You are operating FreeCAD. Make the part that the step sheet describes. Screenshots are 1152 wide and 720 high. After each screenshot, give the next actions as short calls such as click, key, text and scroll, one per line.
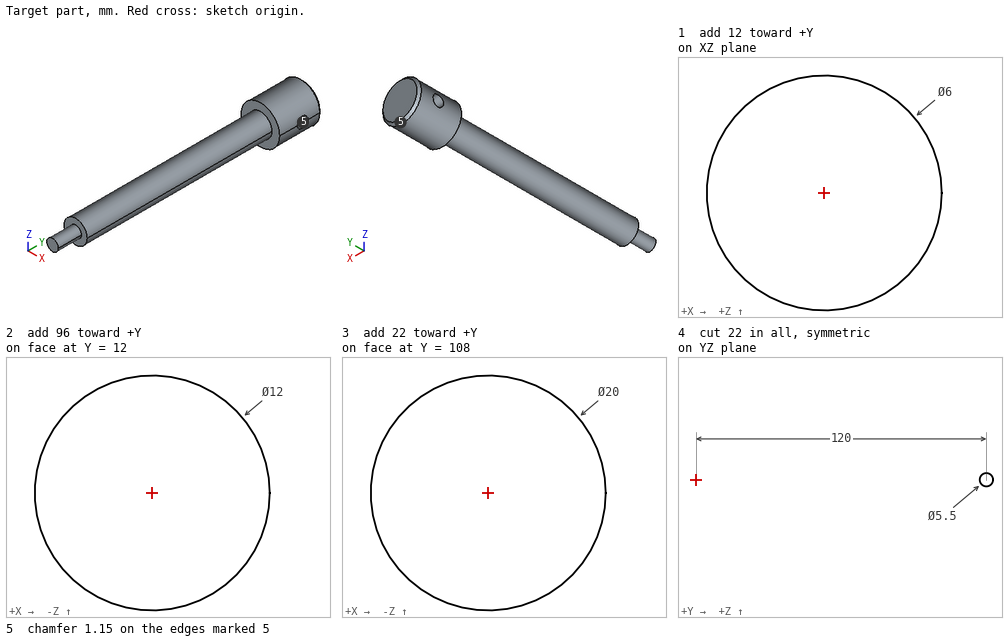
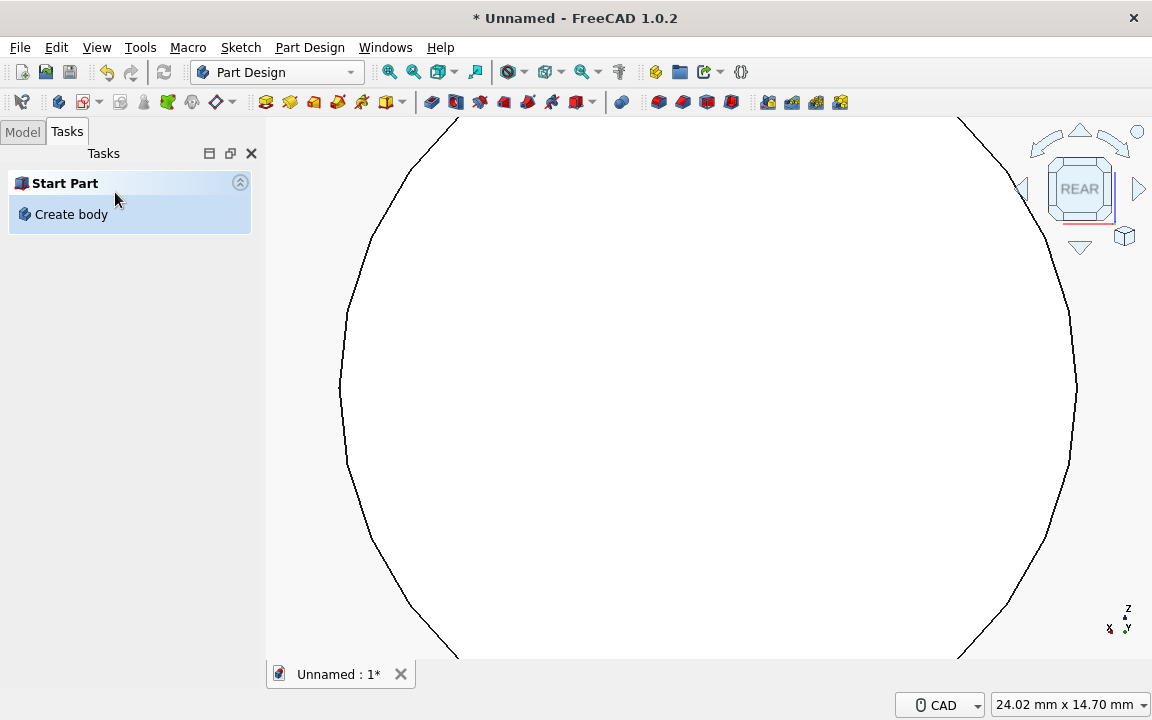
click(390, 72)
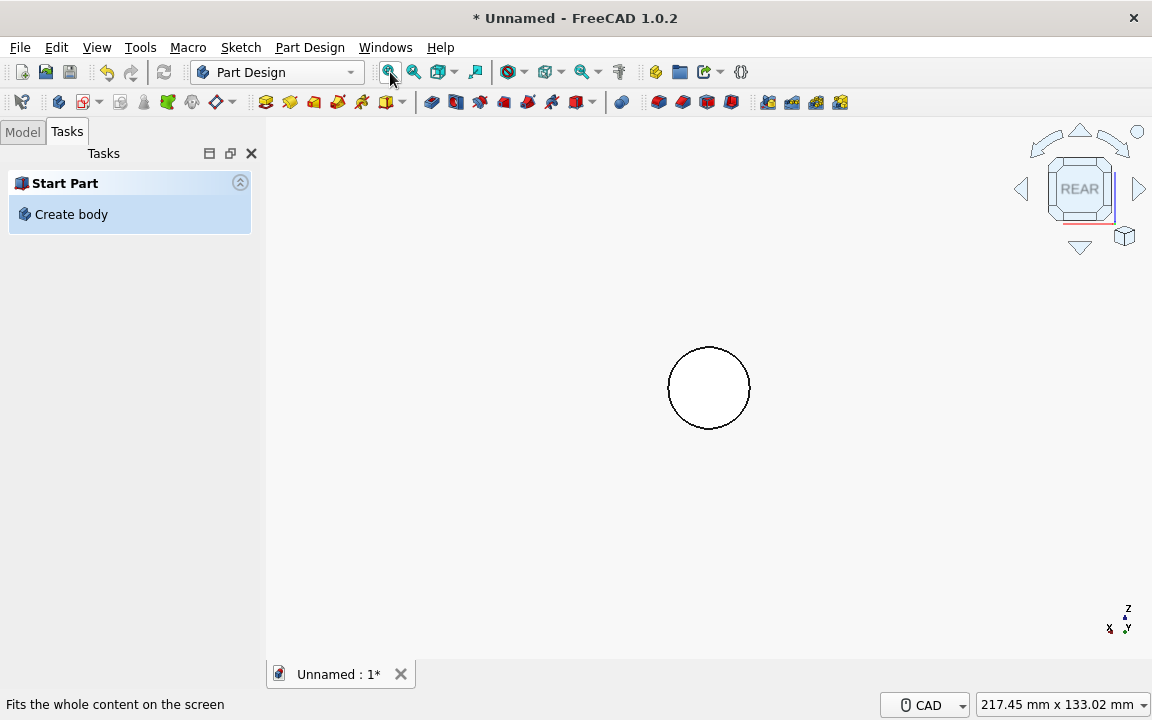
click(84, 102)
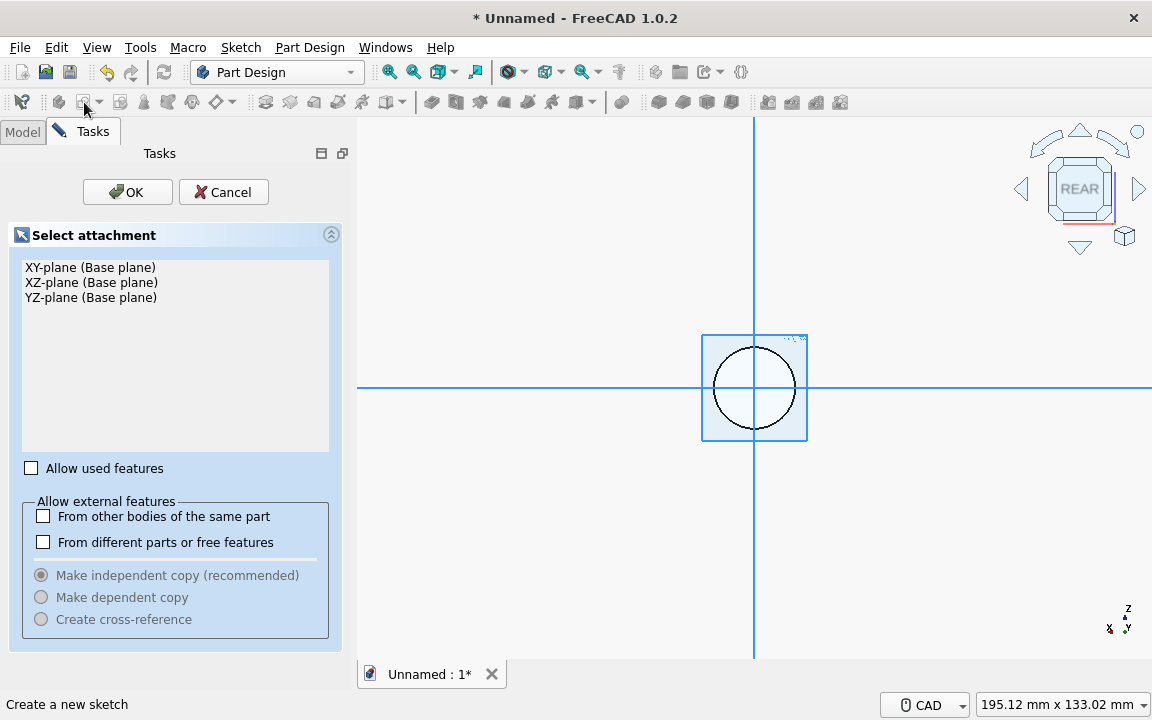
click(82, 298)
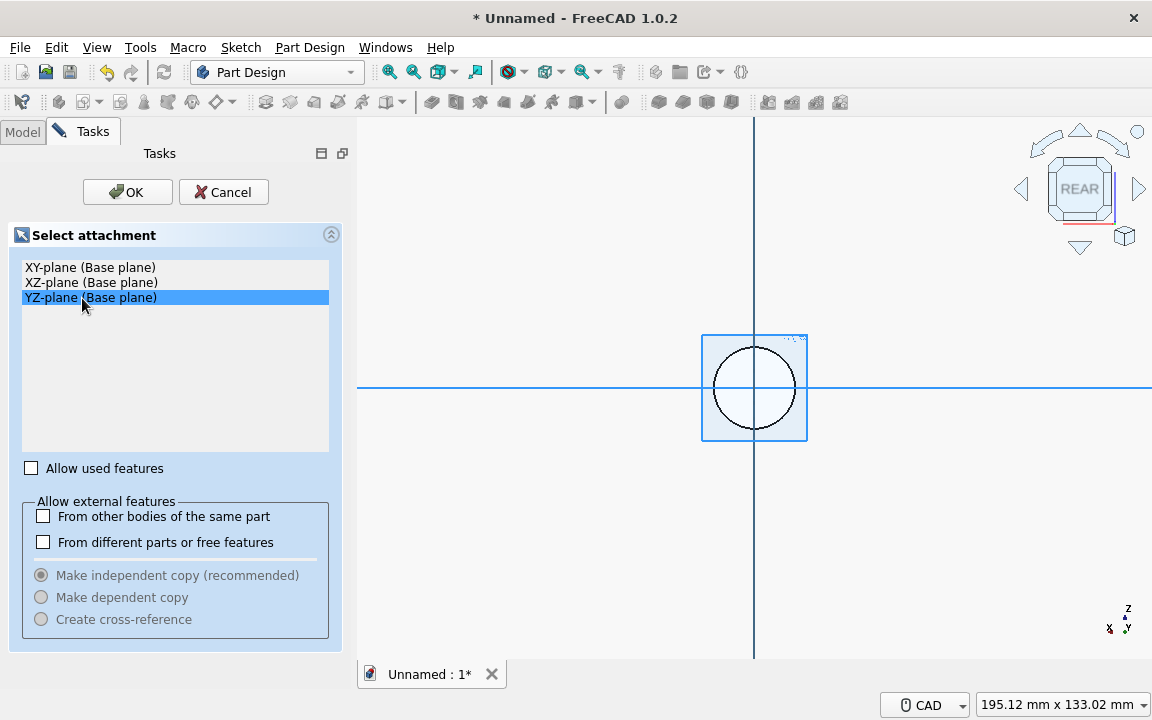
click(128, 192)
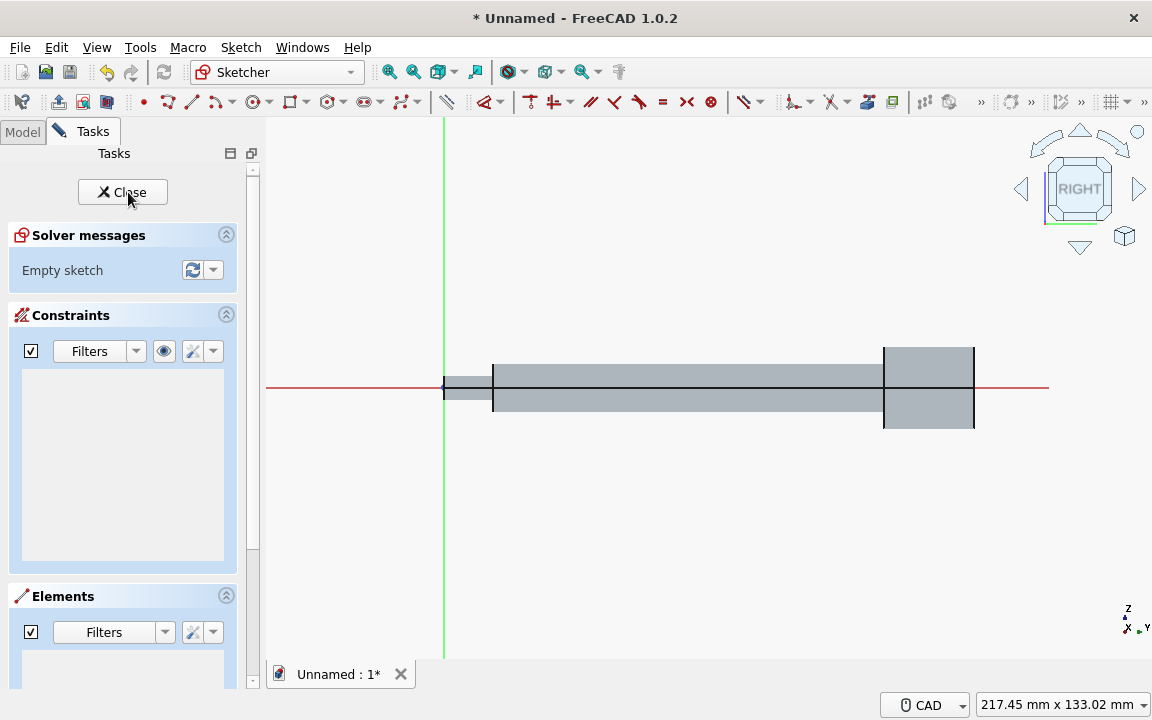
click(108, 102)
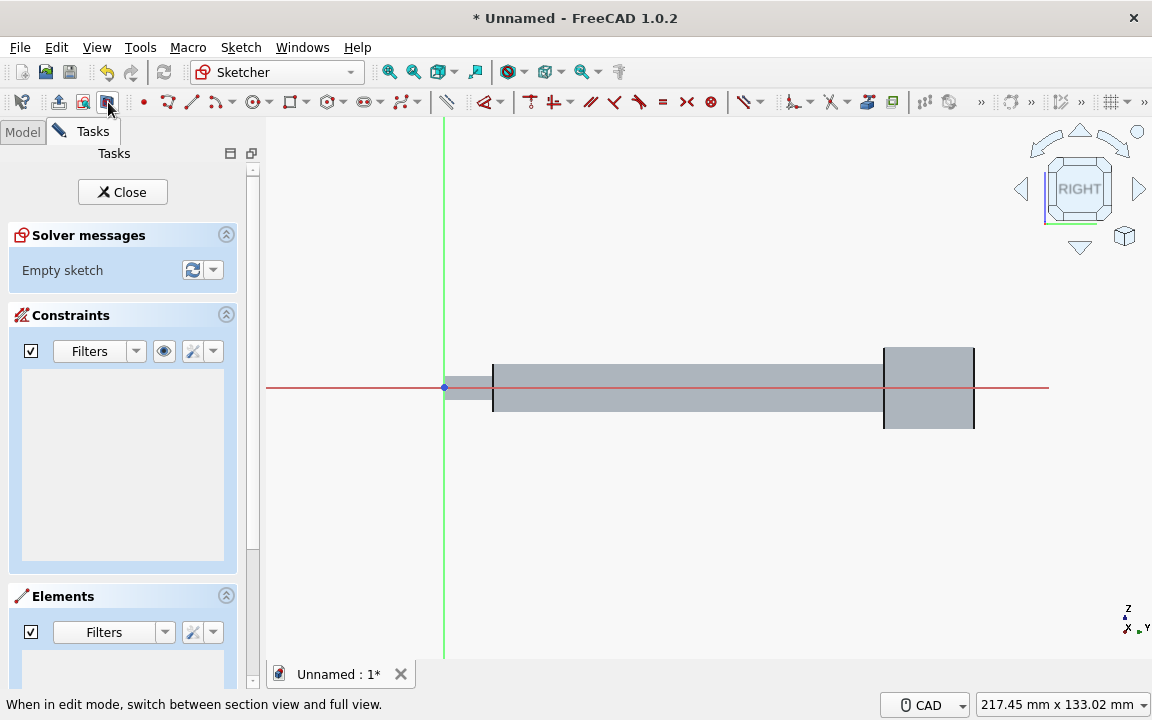
scroll(952, 388, up, 14)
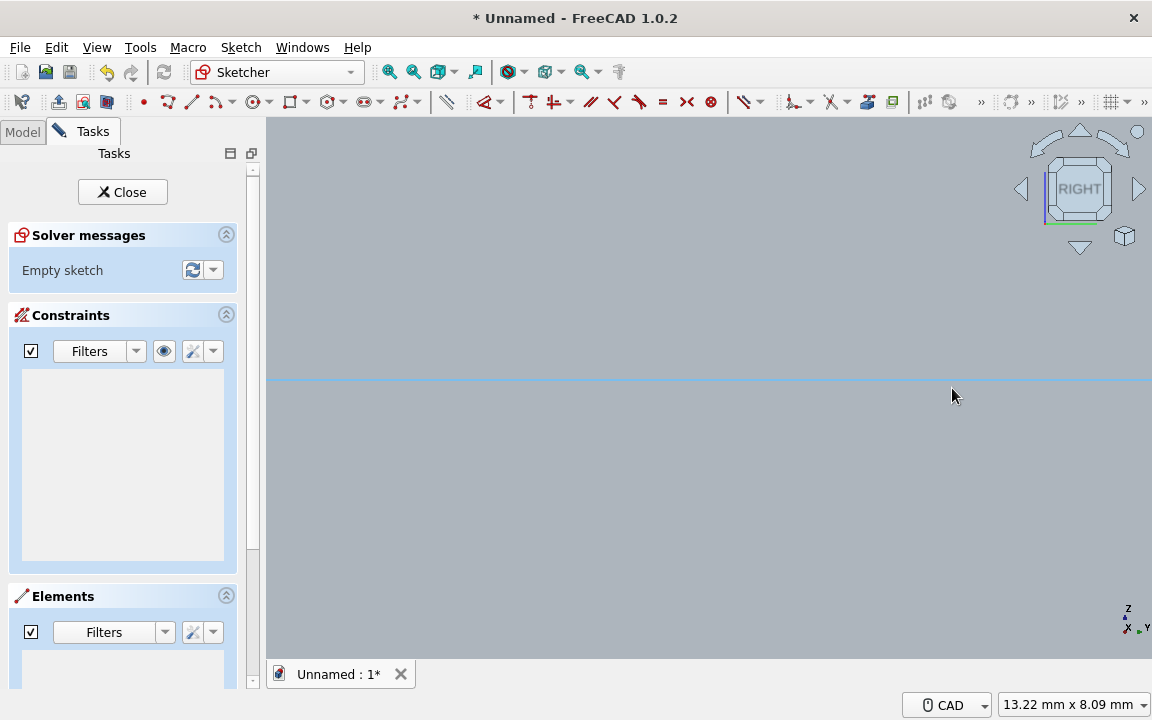
click(254, 102)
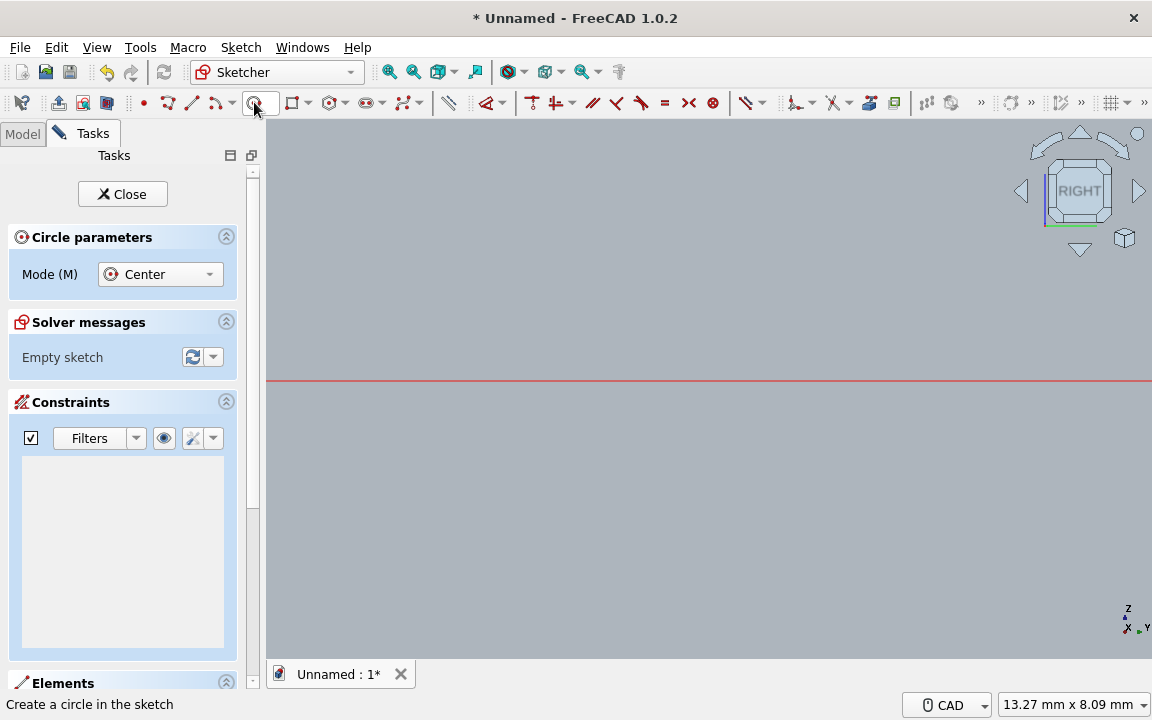
click(629, 381)
move(759, 251)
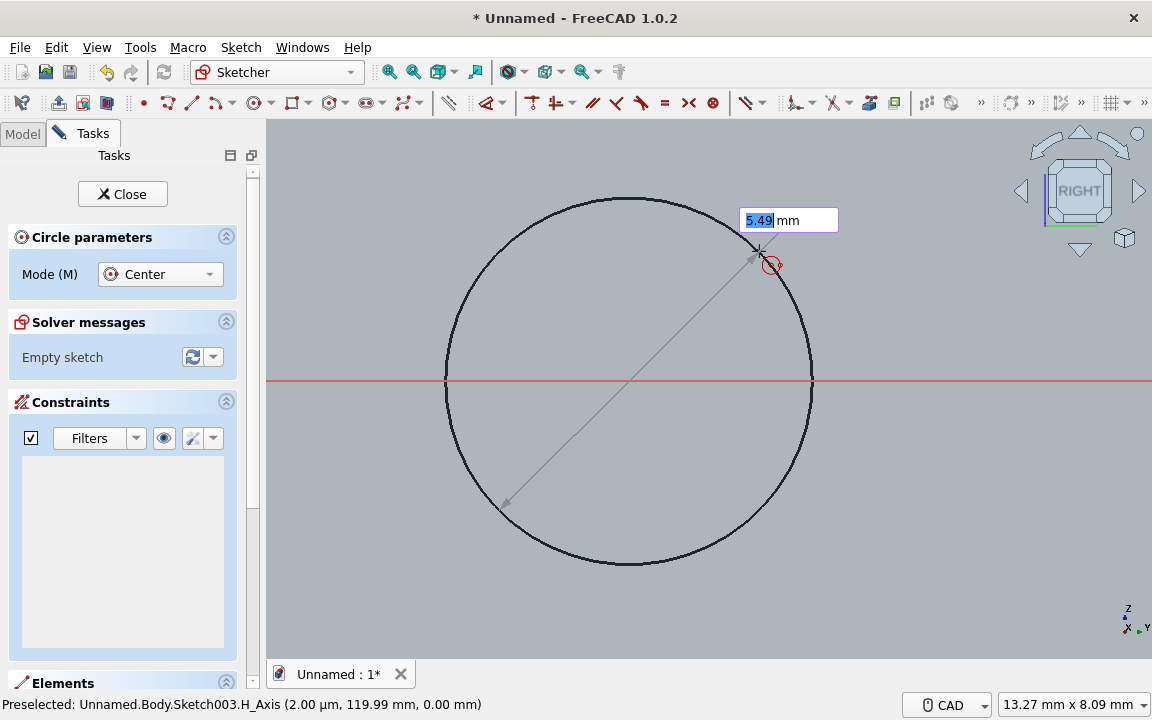
text(5.5)
key(Return)
key(Escape)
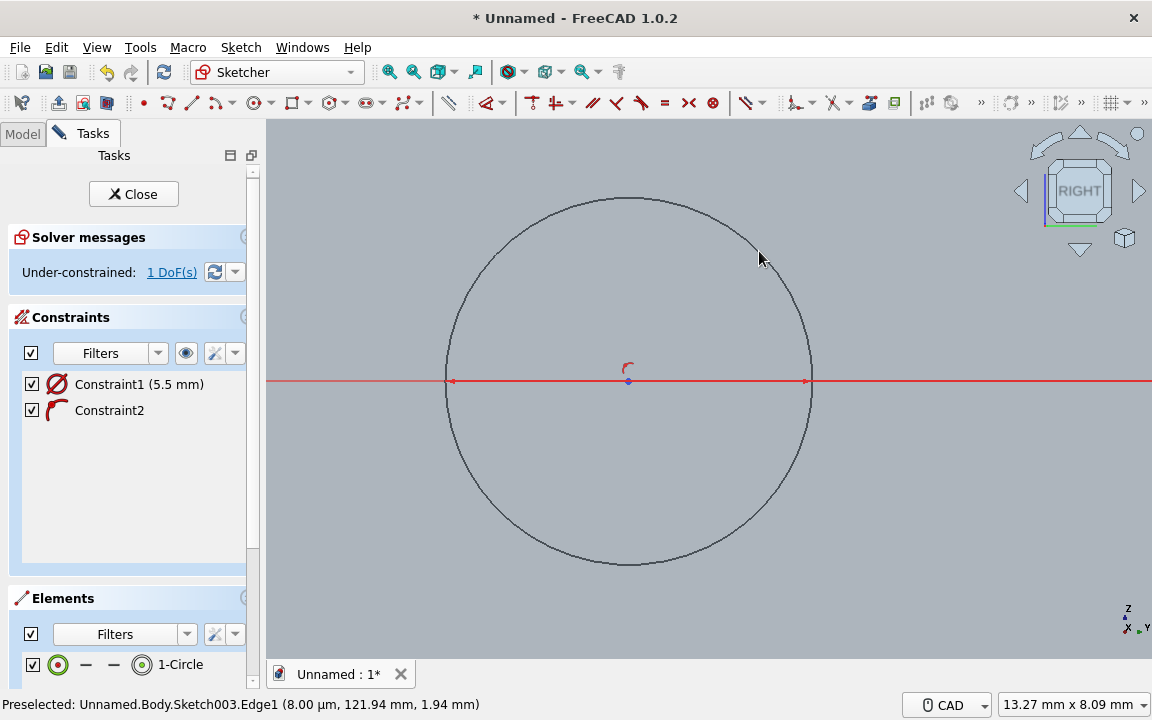
click(486, 104)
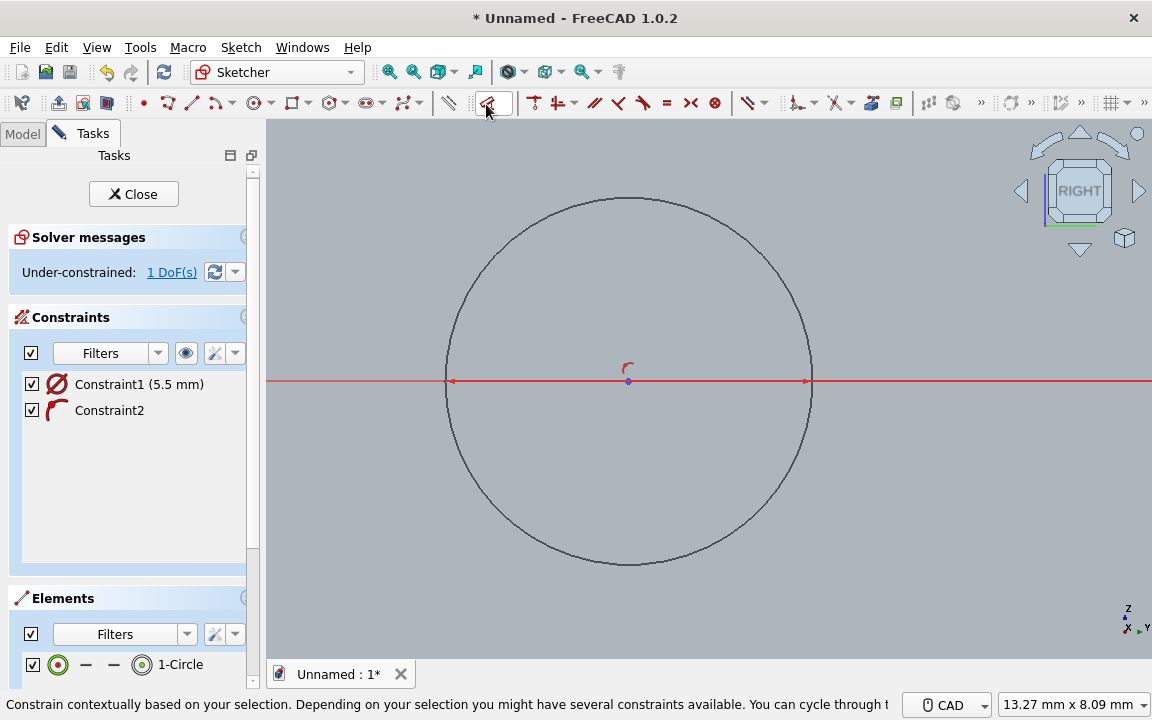
click(629, 381)
click(384, 415)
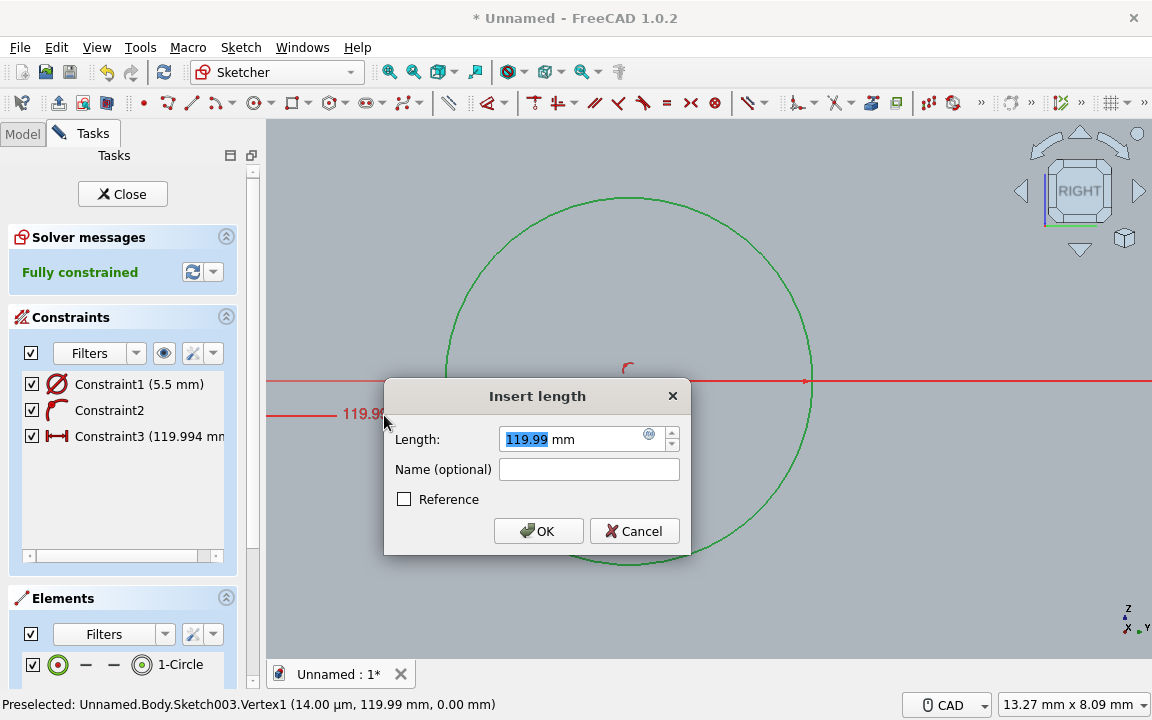
text(120)
key(Return)
key(Escape)